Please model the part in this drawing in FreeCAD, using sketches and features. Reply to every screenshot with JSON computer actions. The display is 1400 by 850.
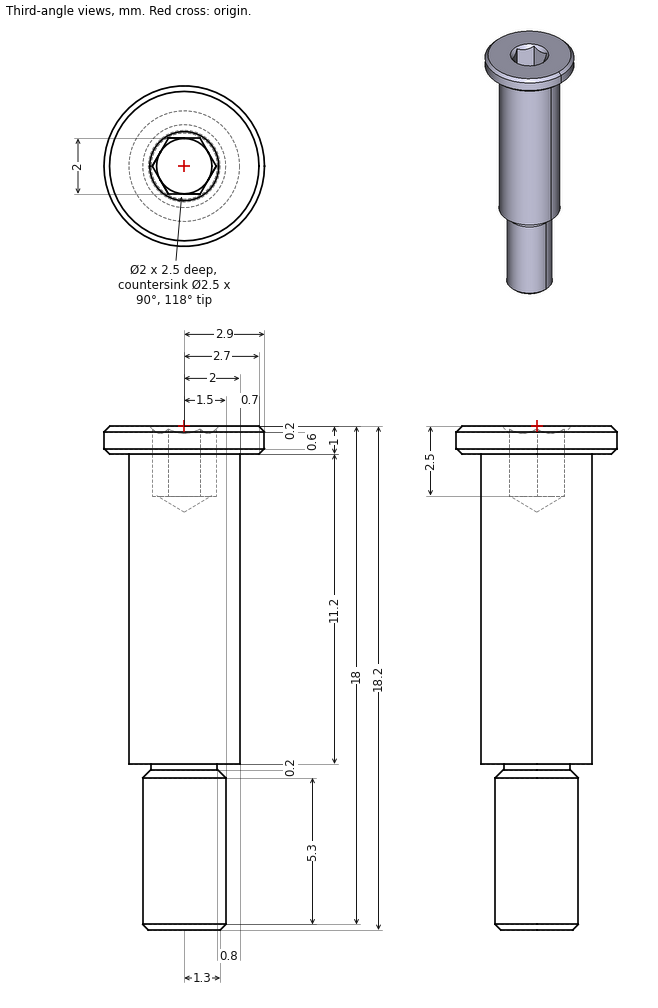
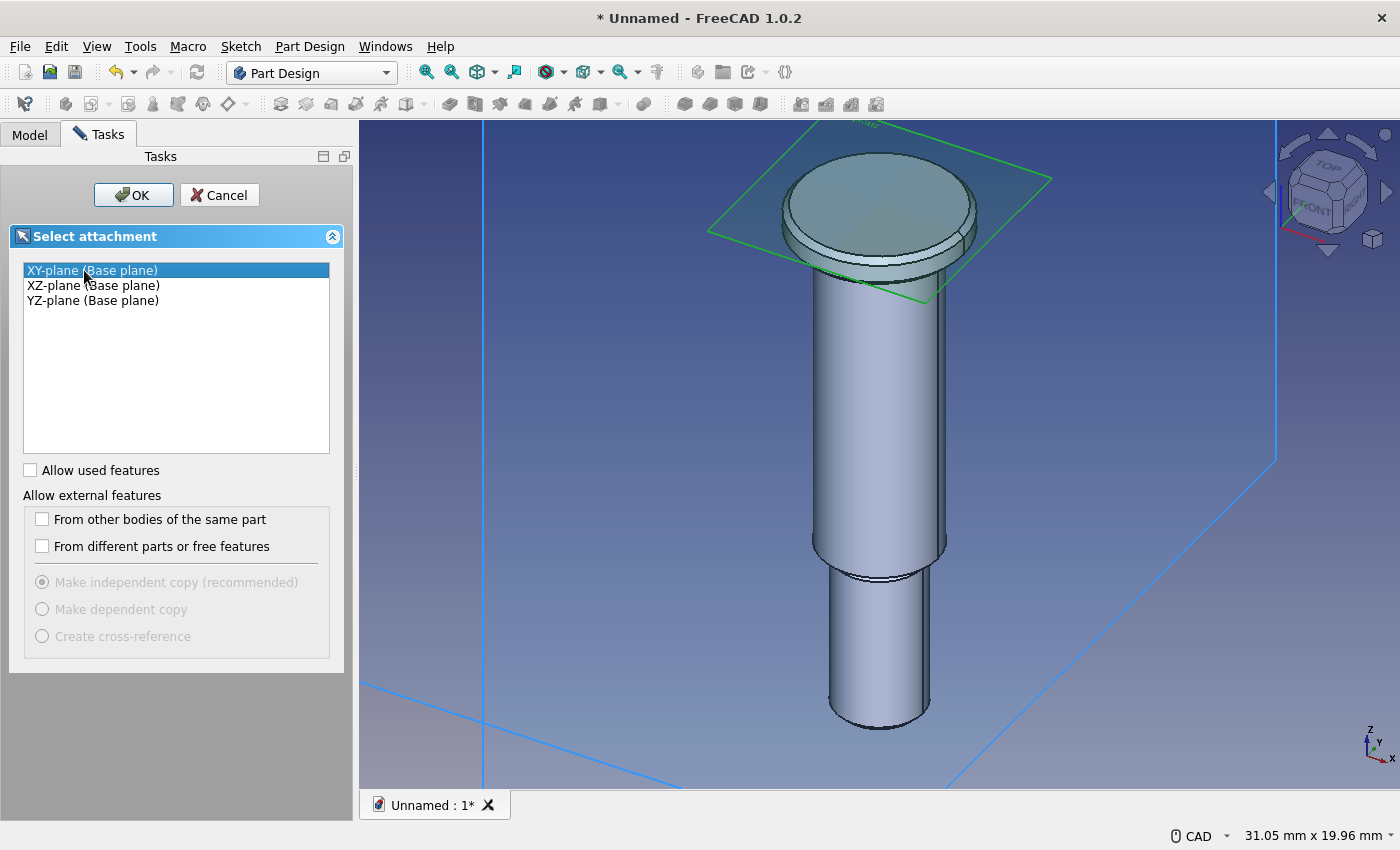
{"action": "left_click", "coordinate": [134, 195]}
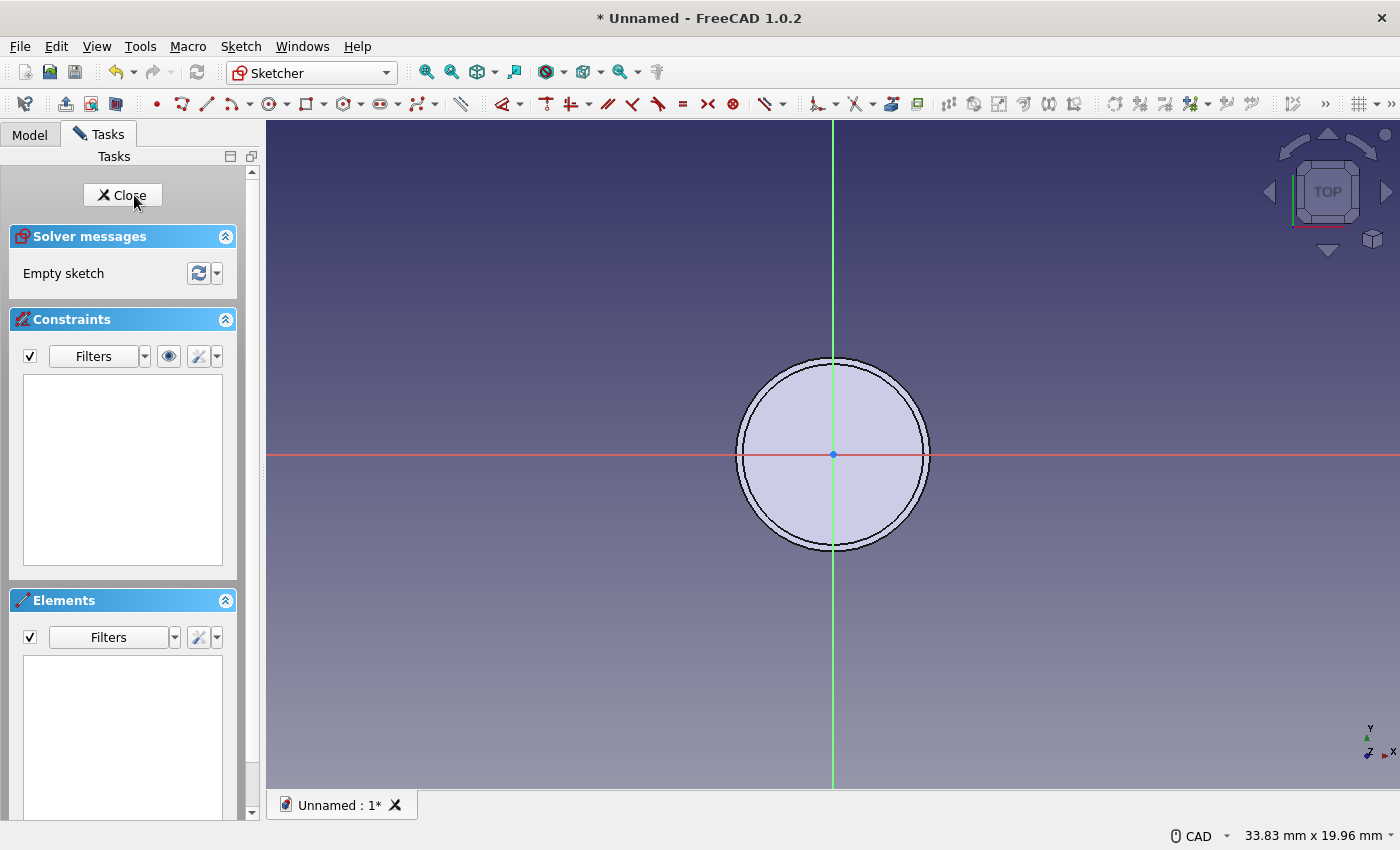
{"action": "scroll", "coordinate": [847, 455], "scroll_direction": "up", "scroll_amount": 9}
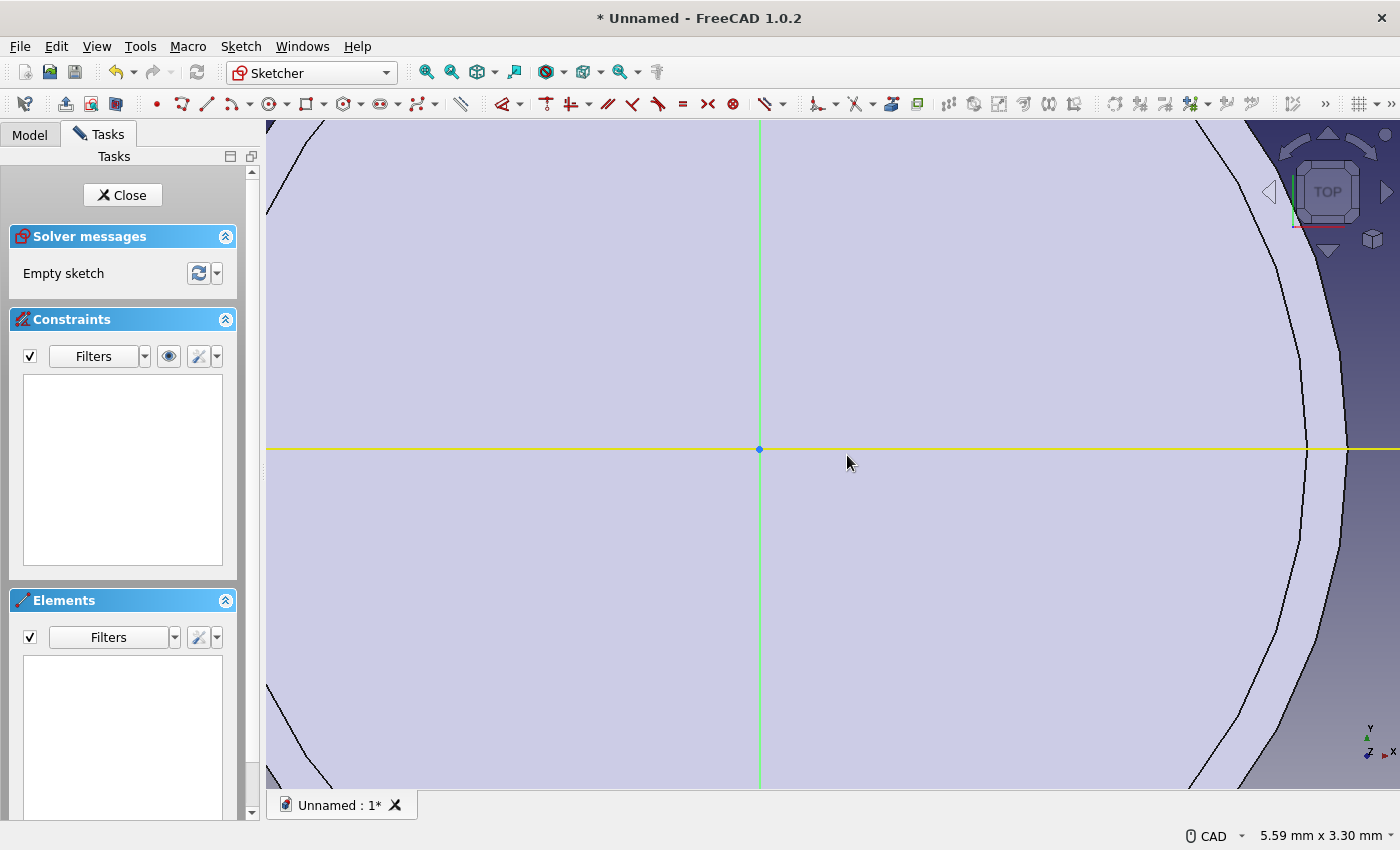
{"action": "left_click", "coordinate": [268, 104]}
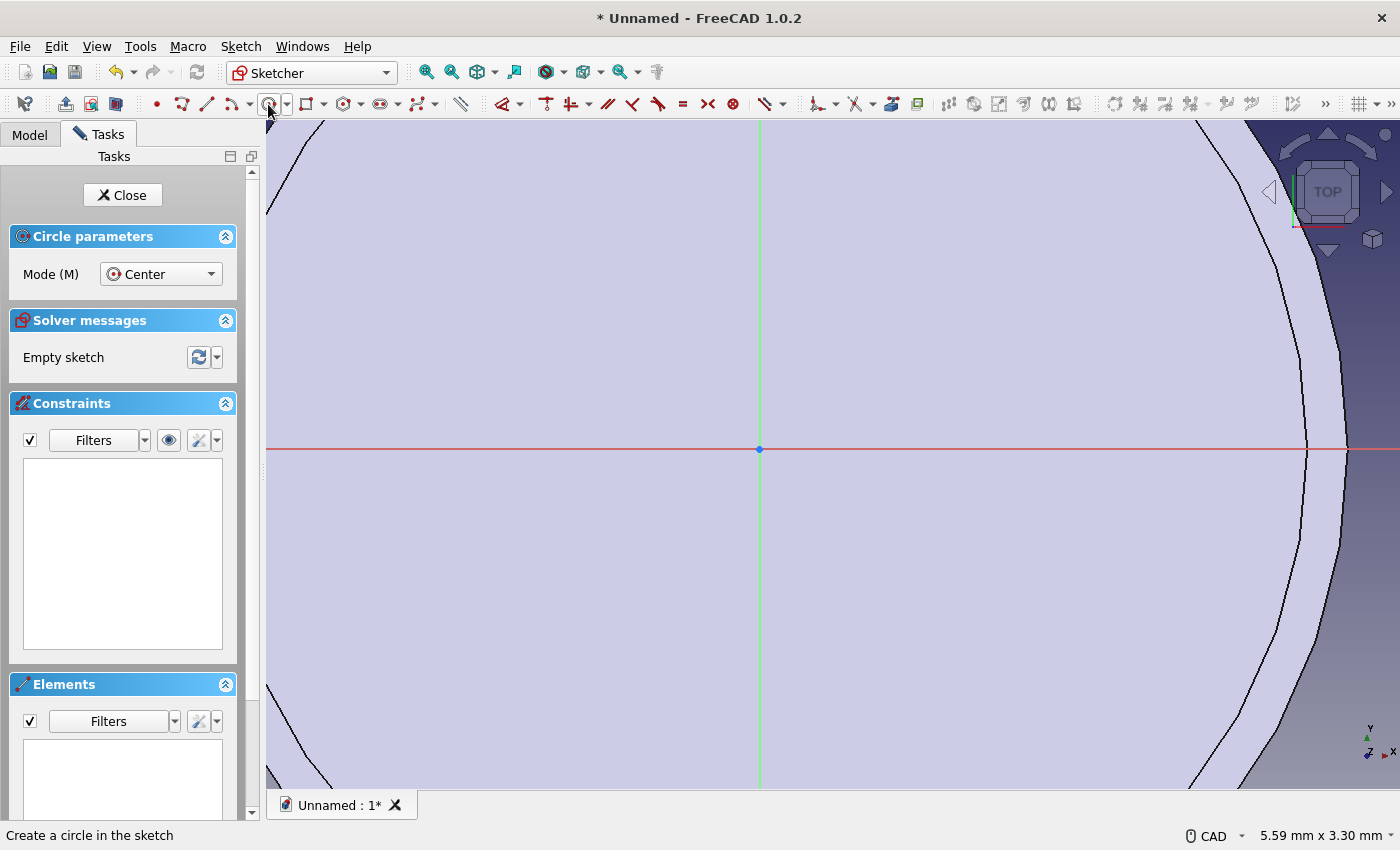
{"action": "left_click", "coordinate": [760, 449]}
{"action": "mouse_move", "coordinate": [903, 306]}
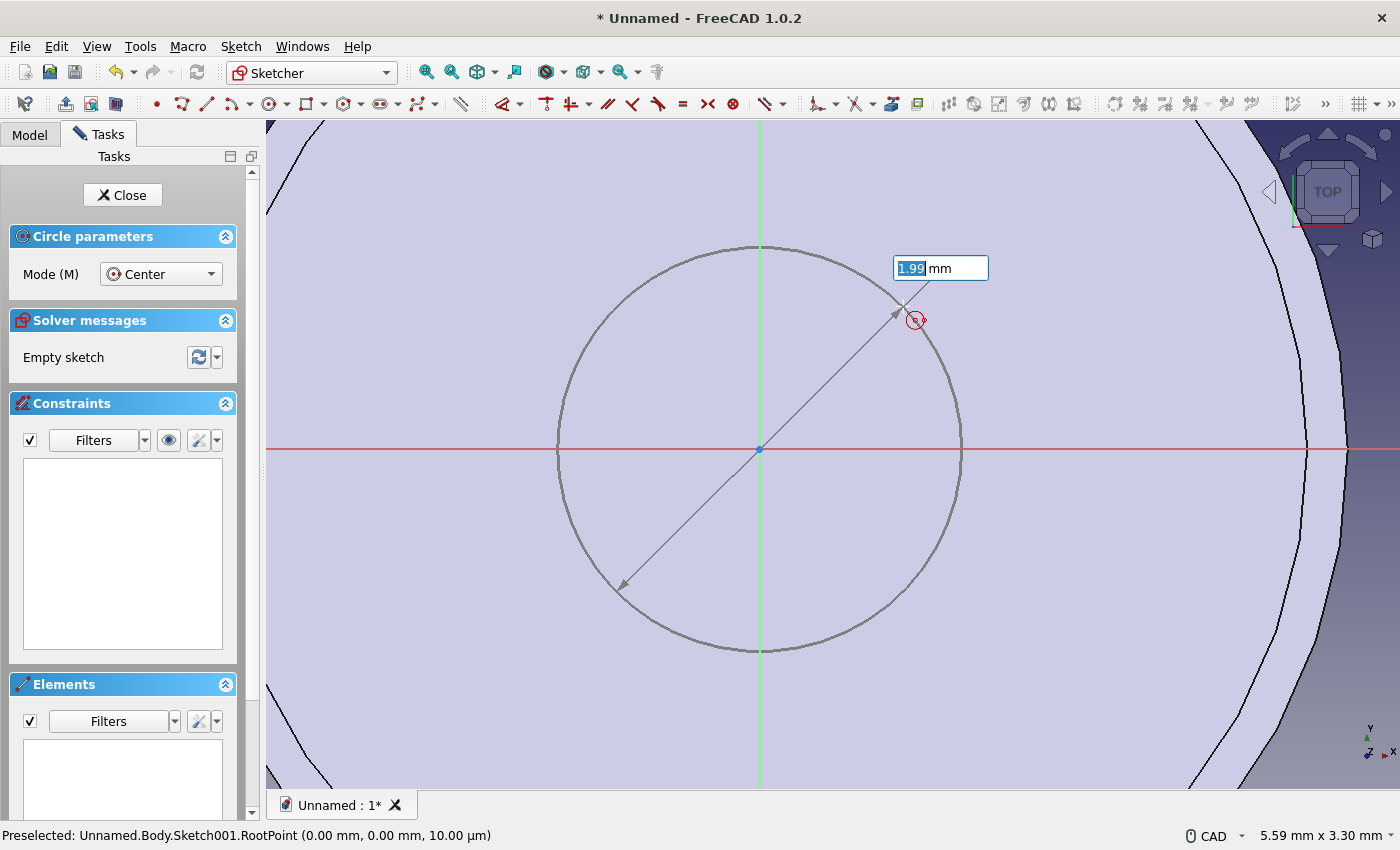
{"action": "type", "text": "2"}
{"action": "key", "text": "Return"}
{"action": "key", "text": "Escape"}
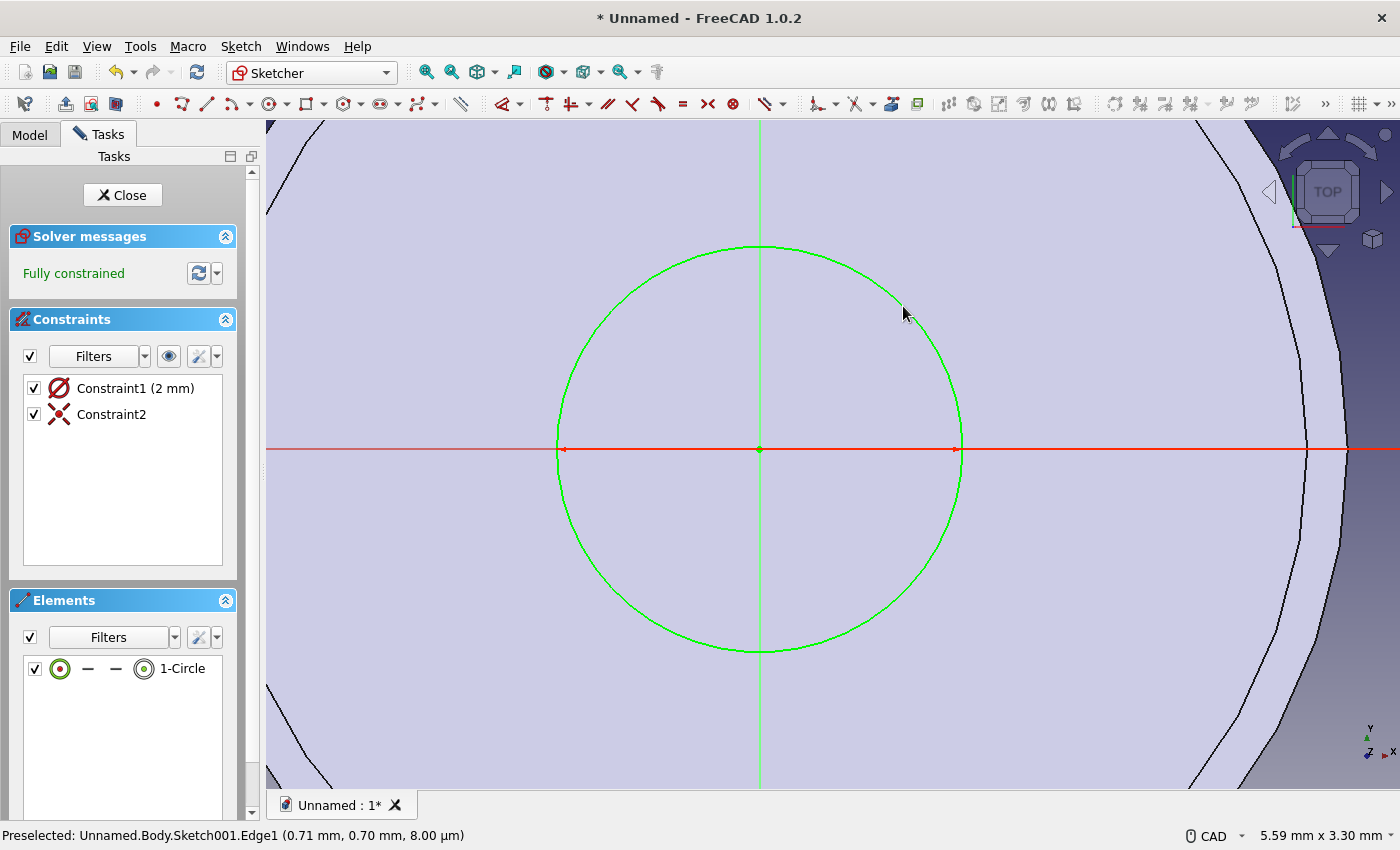
{"action": "left_click", "coordinate": [123, 195]}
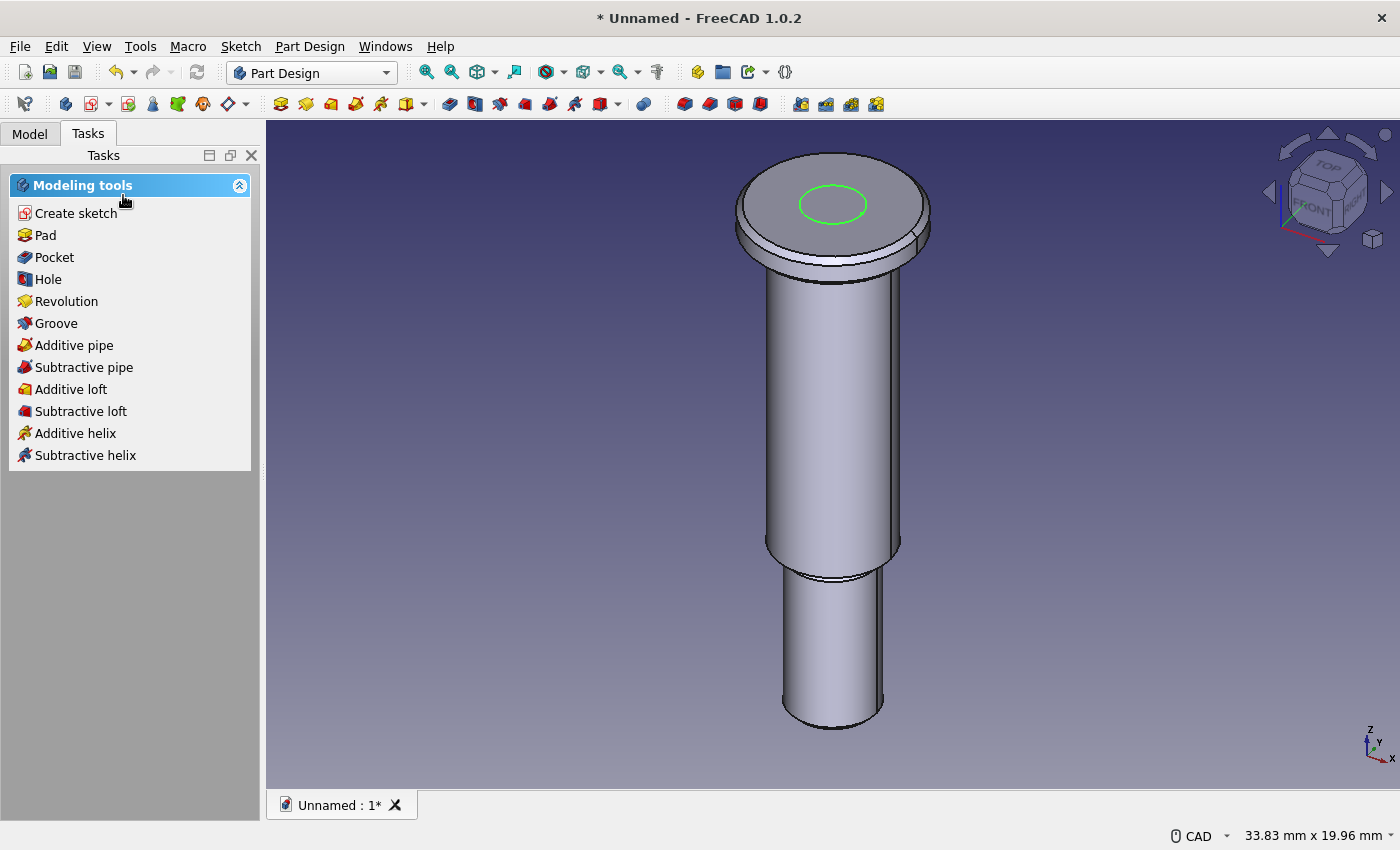
{"action": "left_click", "coordinate": [475, 104]}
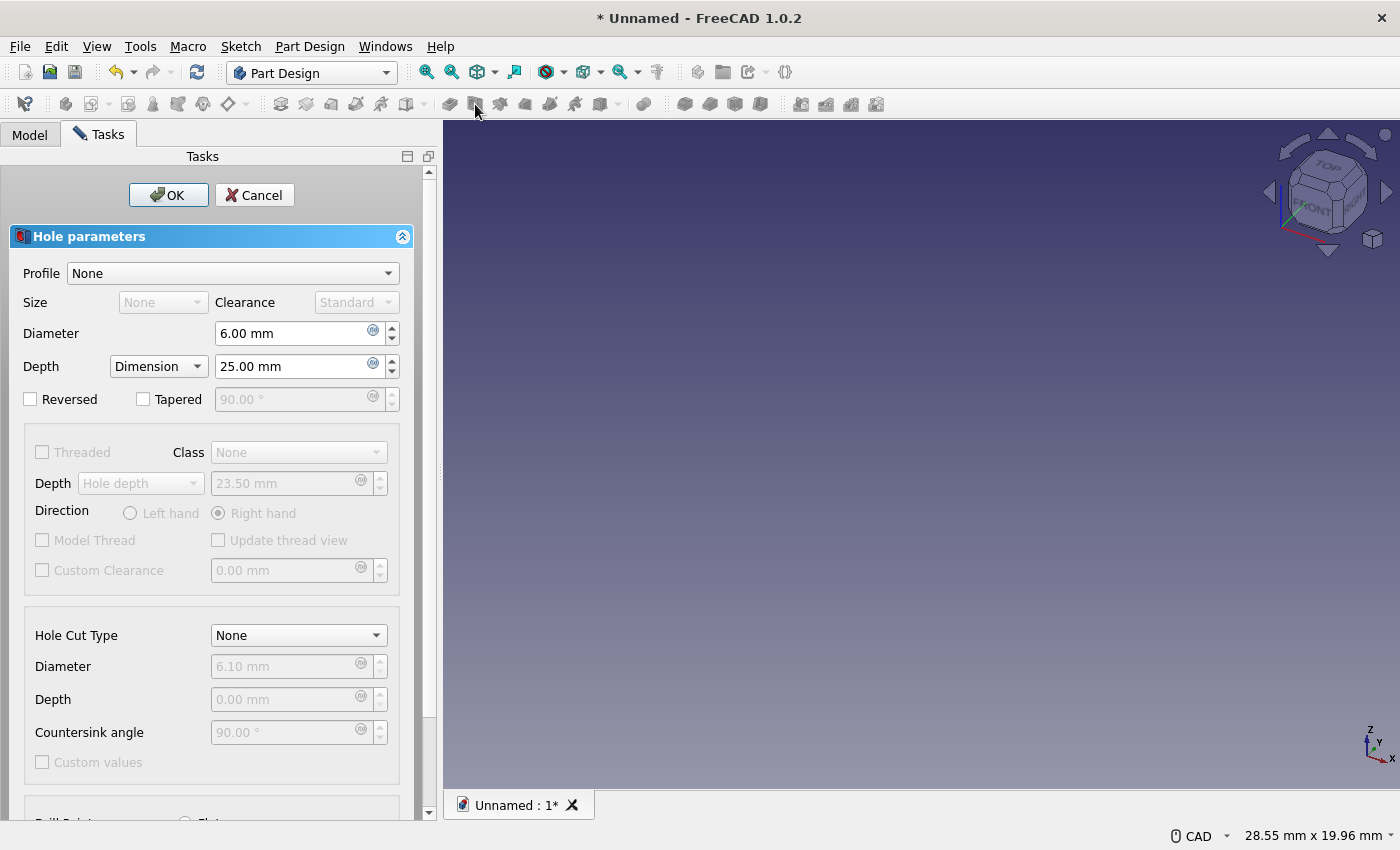
{"action": "triple_click", "coordinate": [300, 334]}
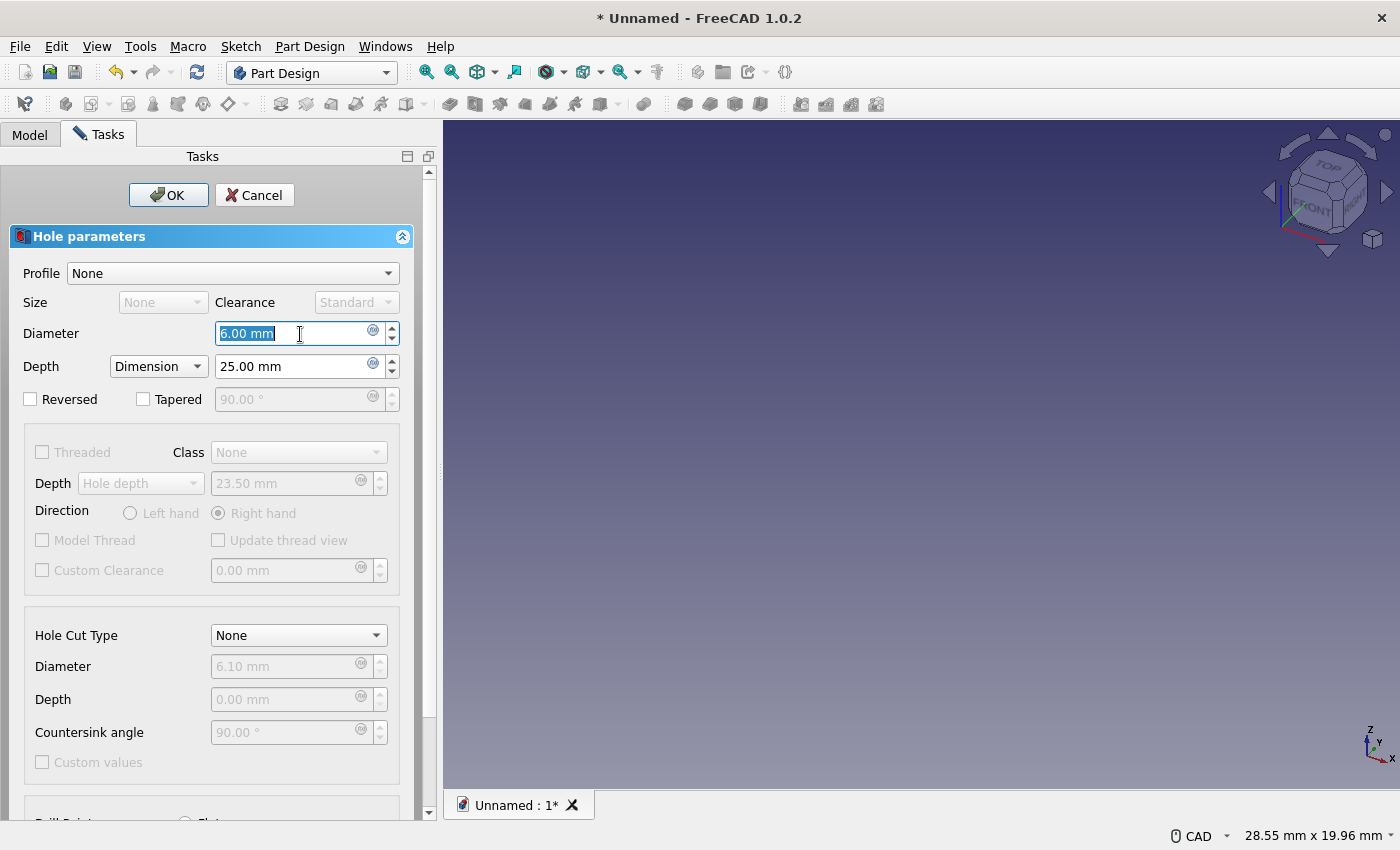
{"action": "type", "text": "2"}
{"action": "key", "text": "Tab"}